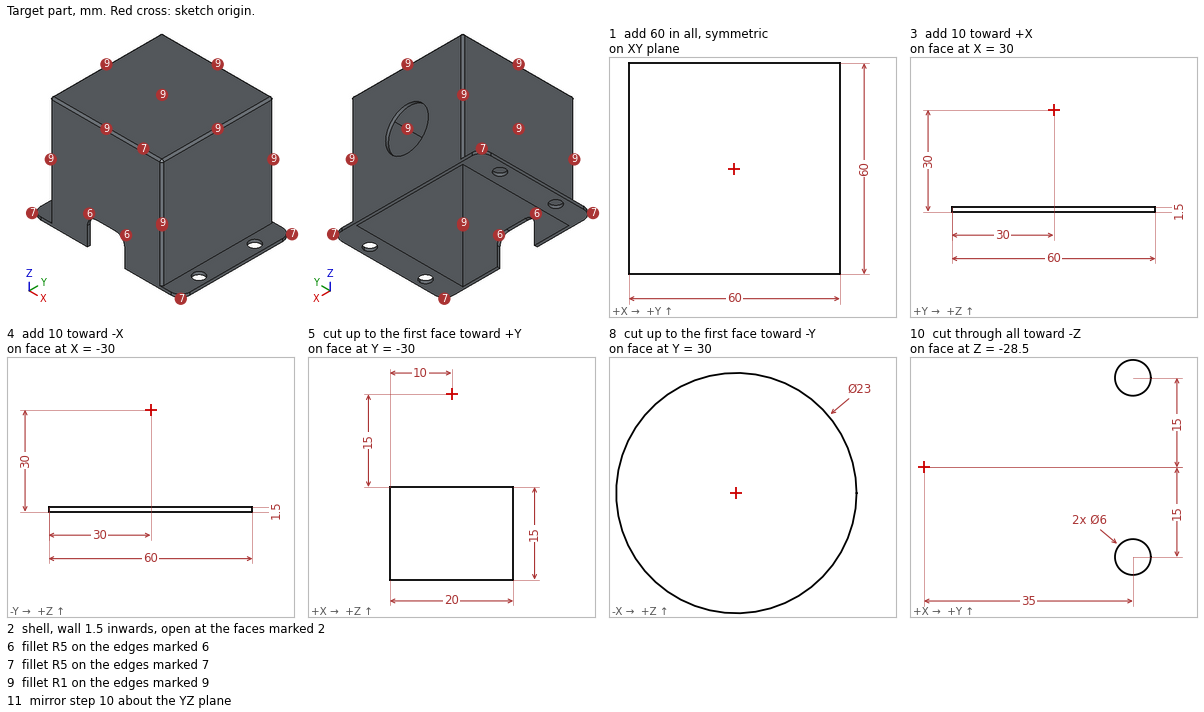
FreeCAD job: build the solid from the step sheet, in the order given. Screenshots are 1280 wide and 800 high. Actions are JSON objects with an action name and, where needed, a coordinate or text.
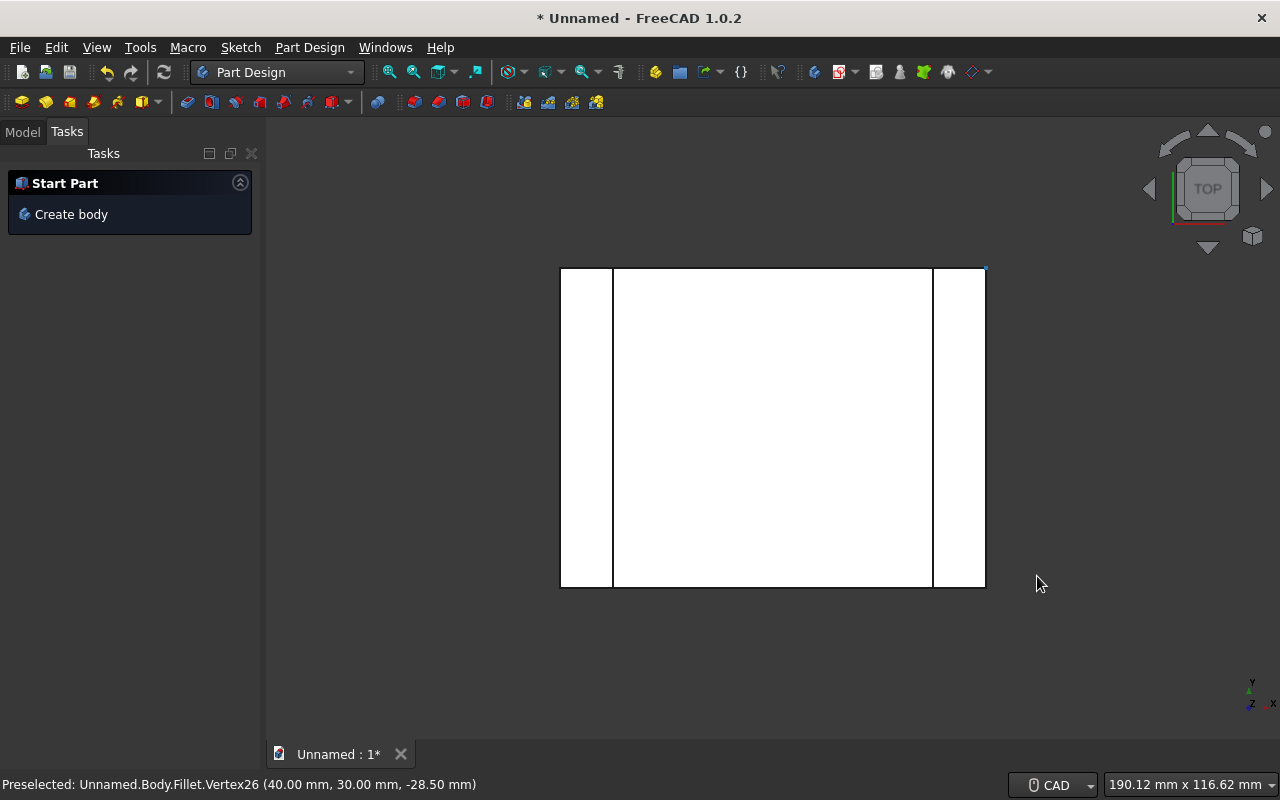
{"action": "scroll", "coordinate": [986, 267], "scroll_direction": "up", "scroll_amount": 9}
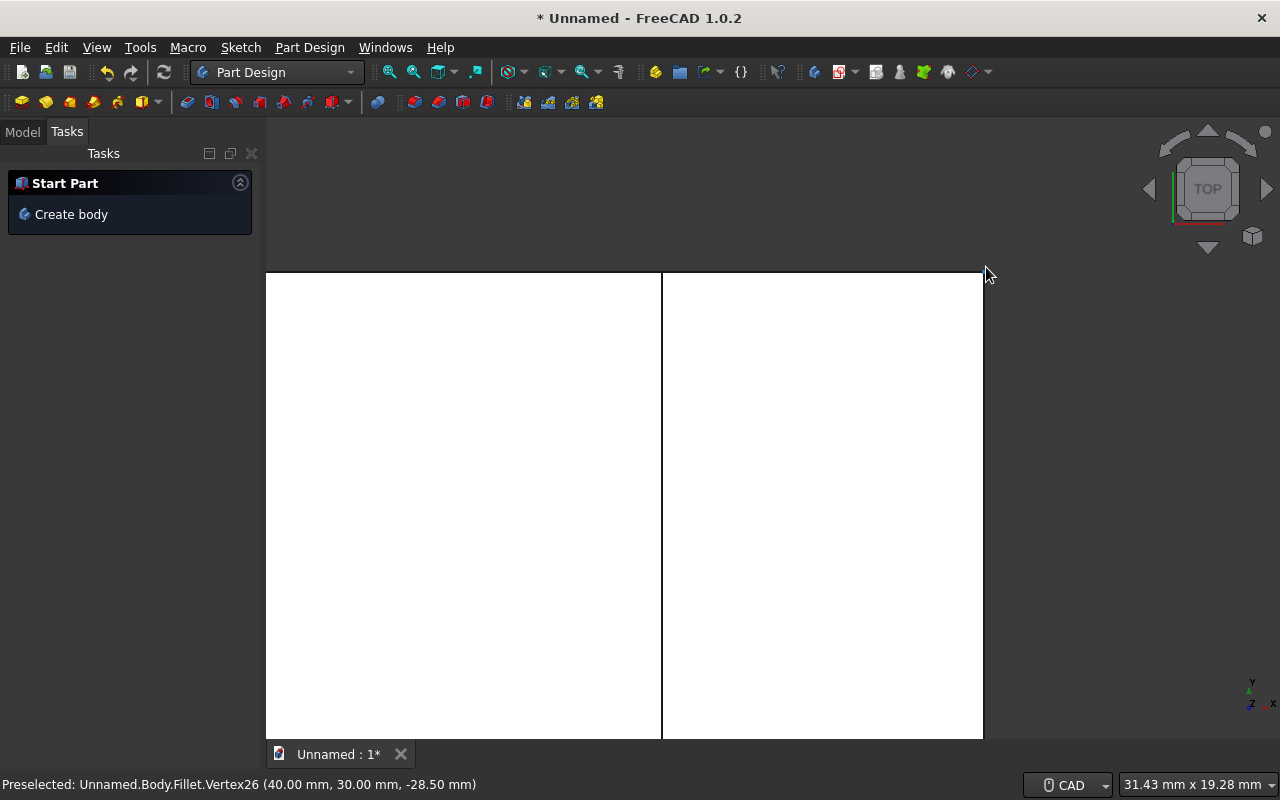
{"action": "key", "text": "v f"}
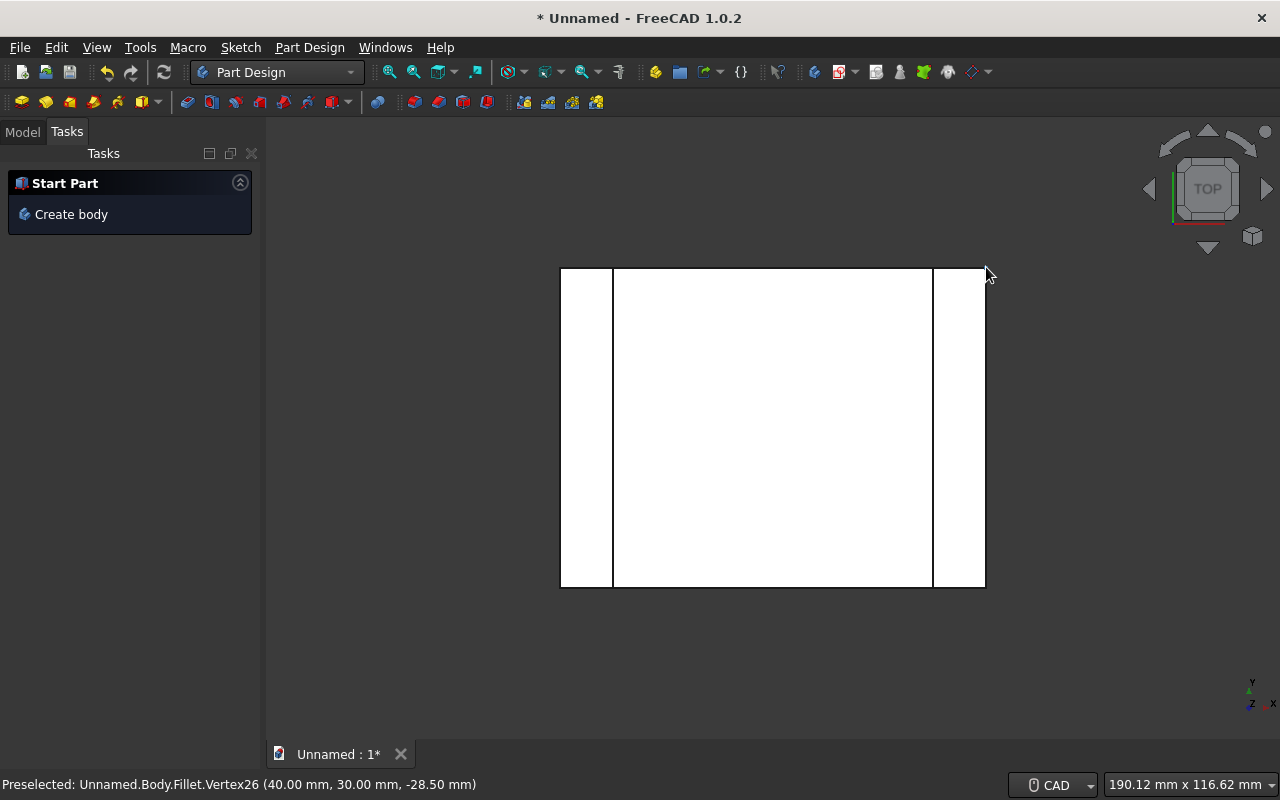
{"action": "key", "text": "1"}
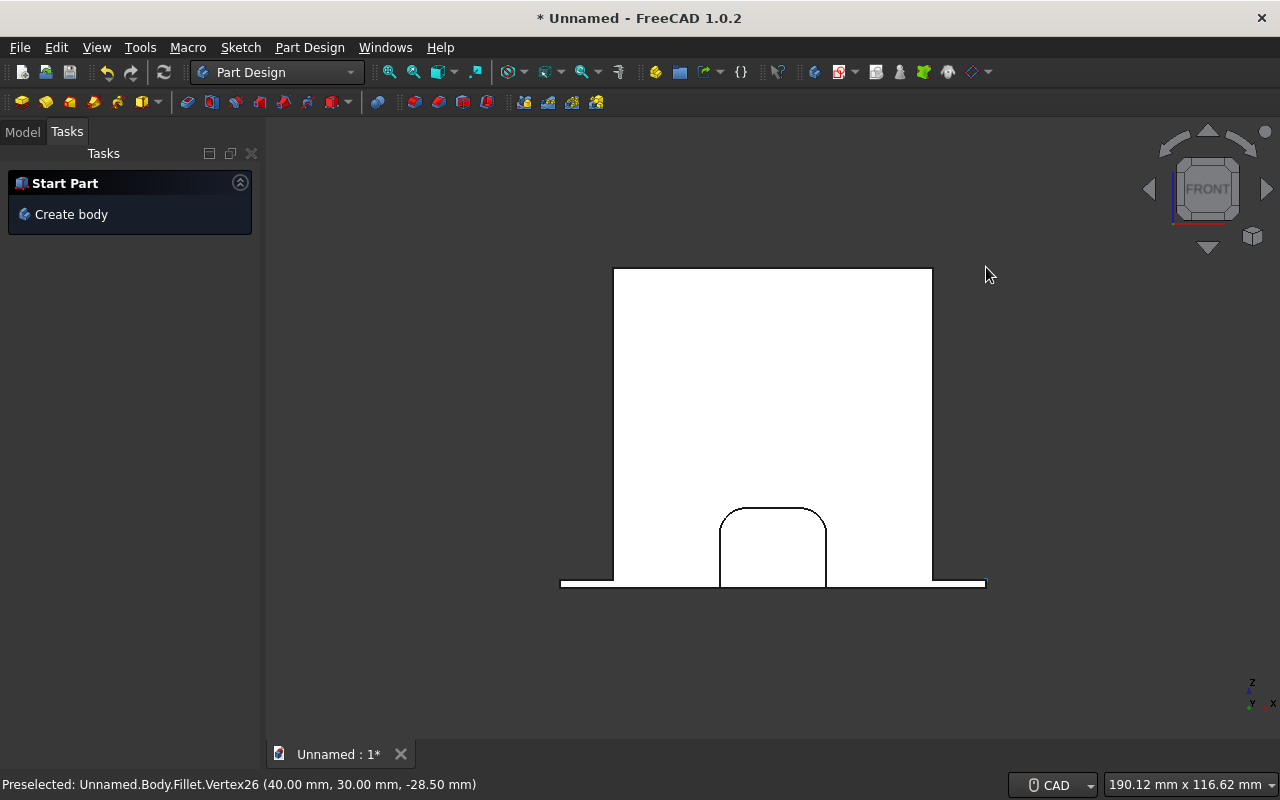
{"action": "scroll", "coordinate": [986, 583], "scroll_direction": "up", "scroll_amount": 9}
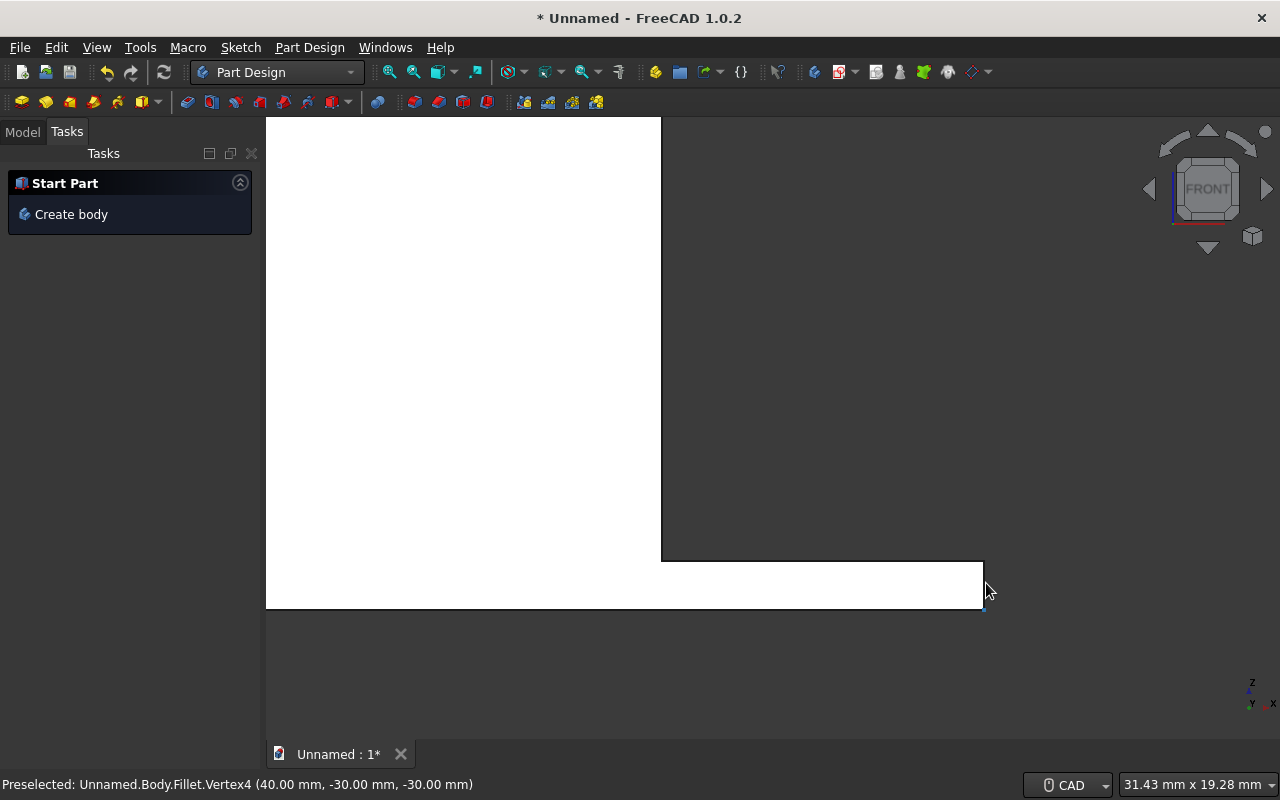
{"action": "left_click", "coordinate": [984, 584]}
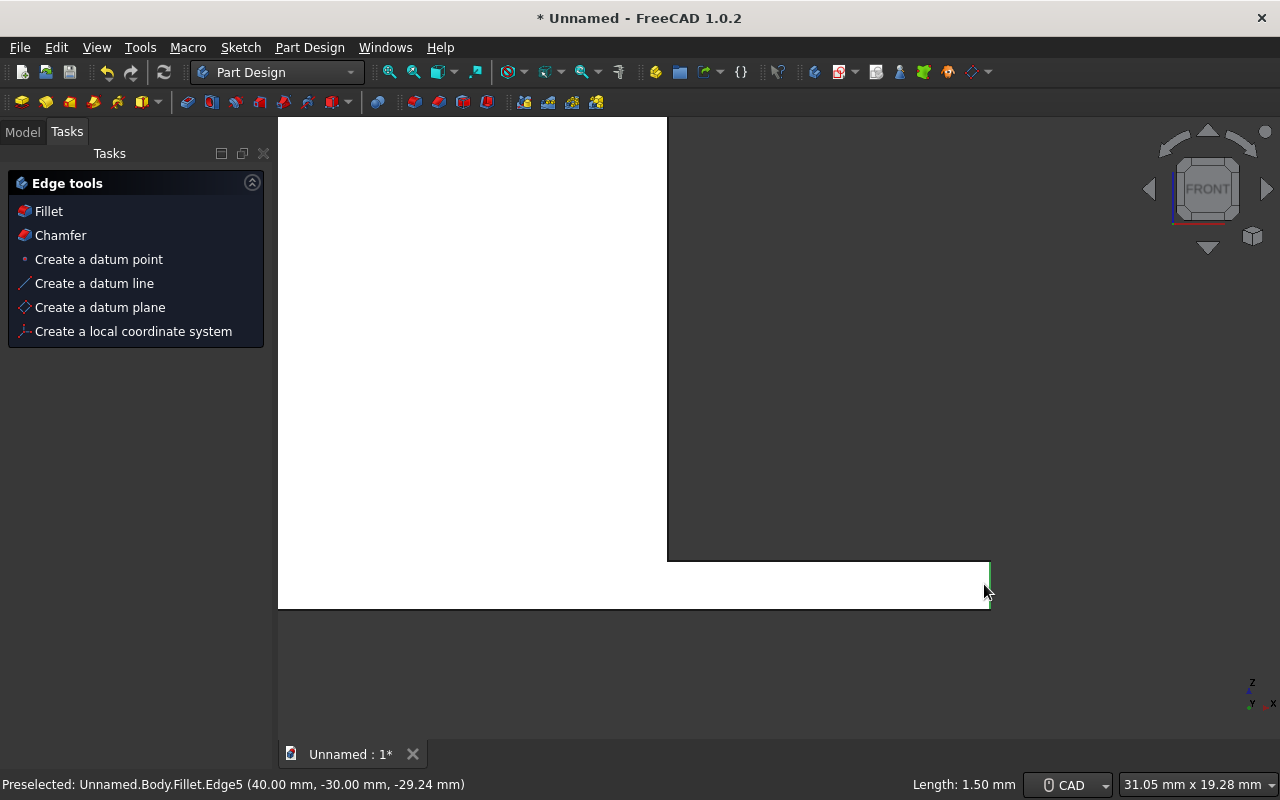
{"action": "key", "text": "v f"}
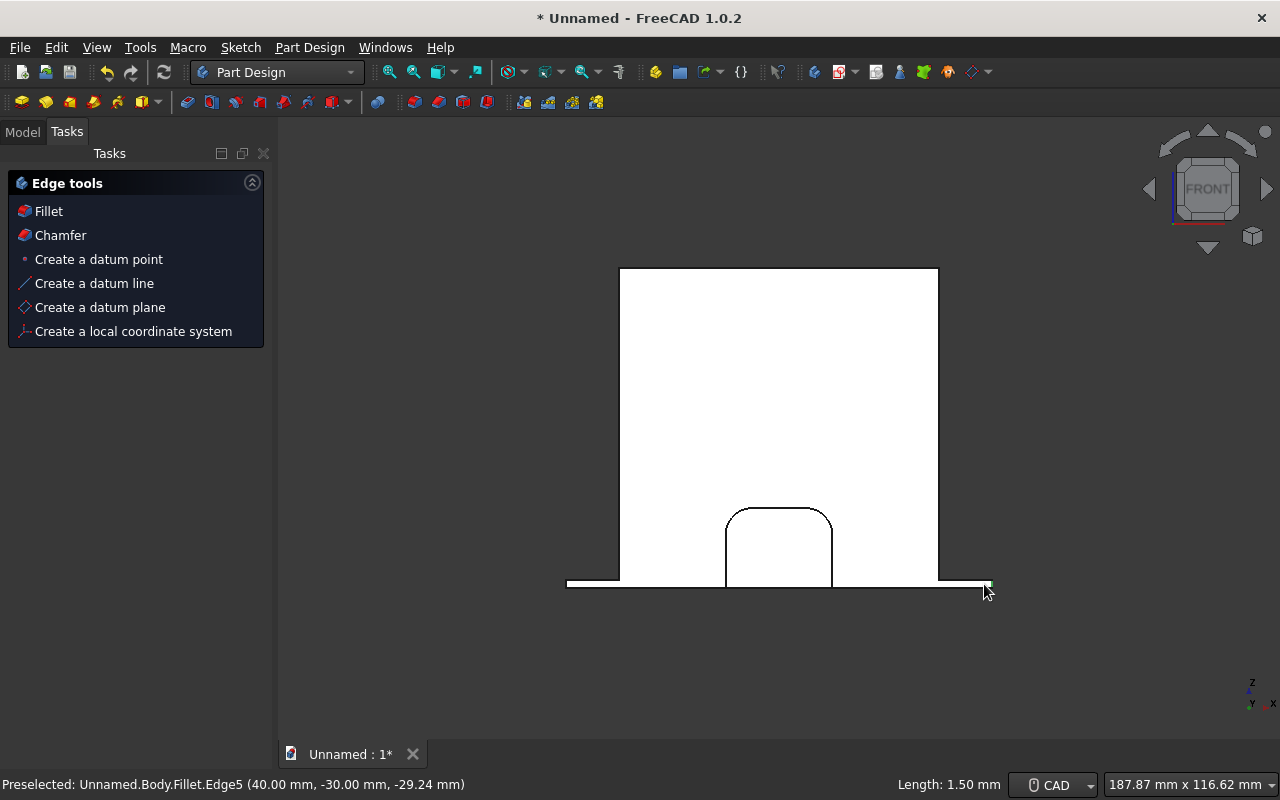
{"action": "key", "text": "3"}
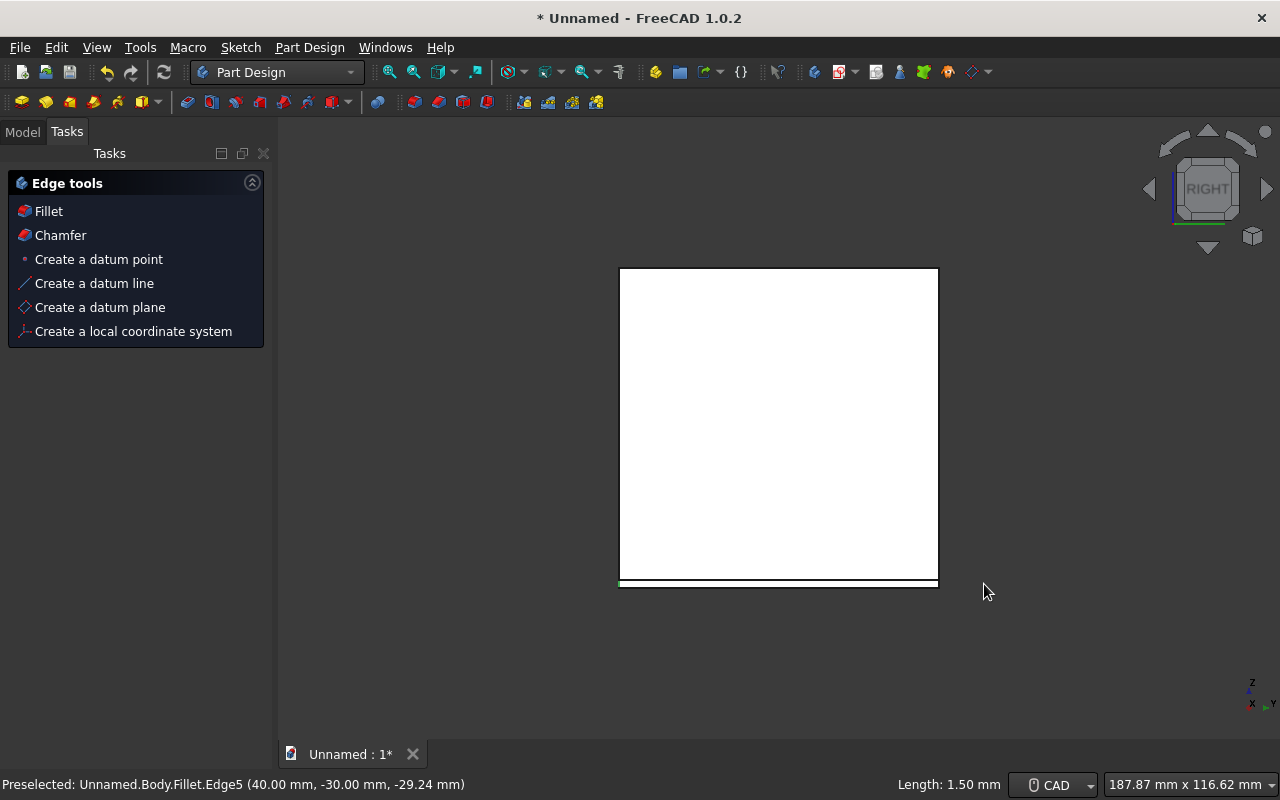
{"action": "scroll", "coordinate": [939, 583], "scroll_direction": "up", "scroll_amount": 9}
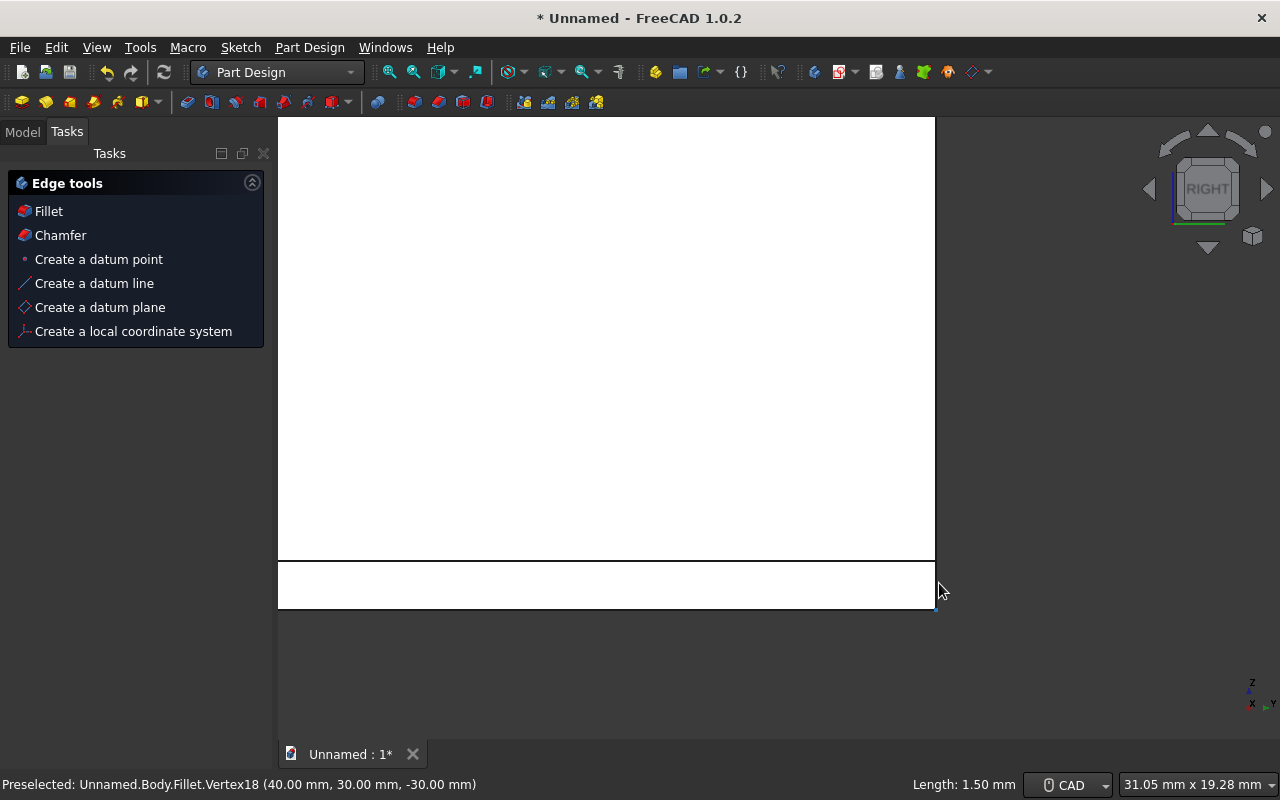
{"action": "left_click", "coordinate": [936, 584], "text": "ctrl"}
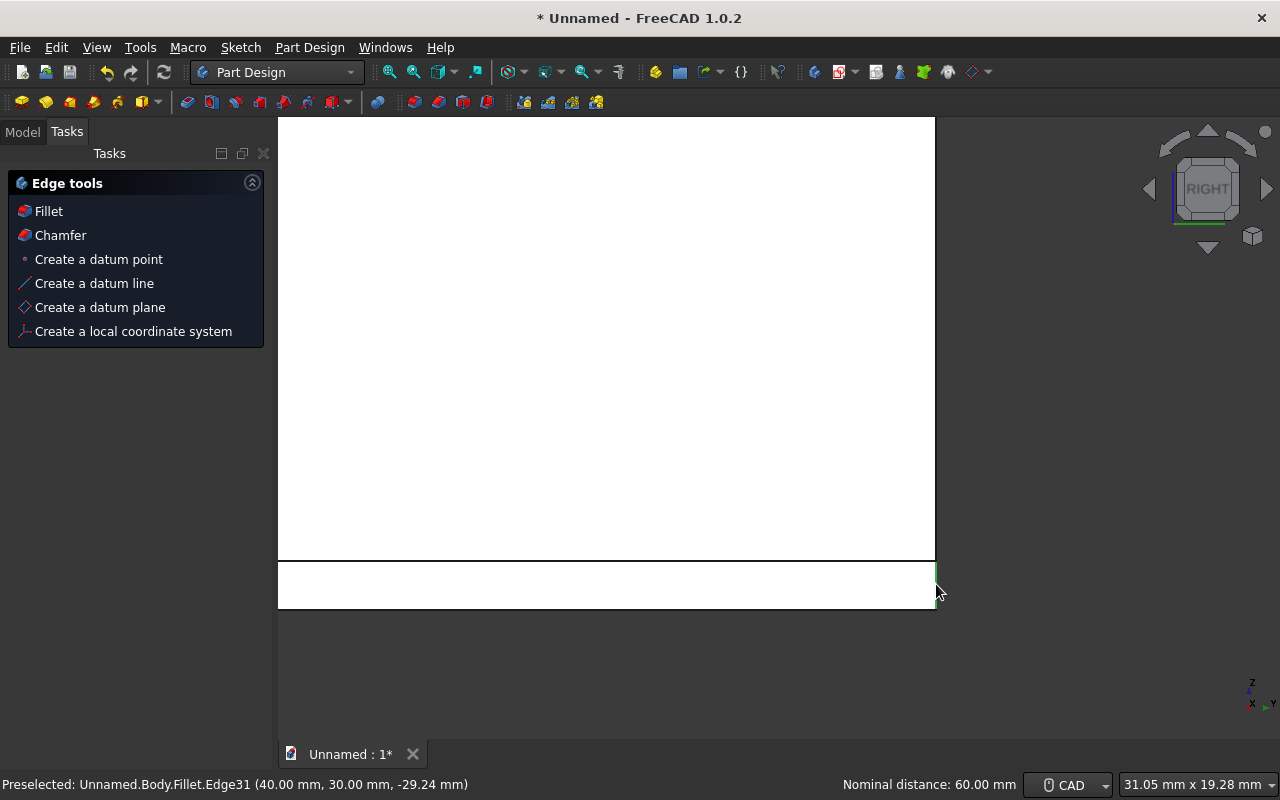
{"action": "key", "text": "v f"}